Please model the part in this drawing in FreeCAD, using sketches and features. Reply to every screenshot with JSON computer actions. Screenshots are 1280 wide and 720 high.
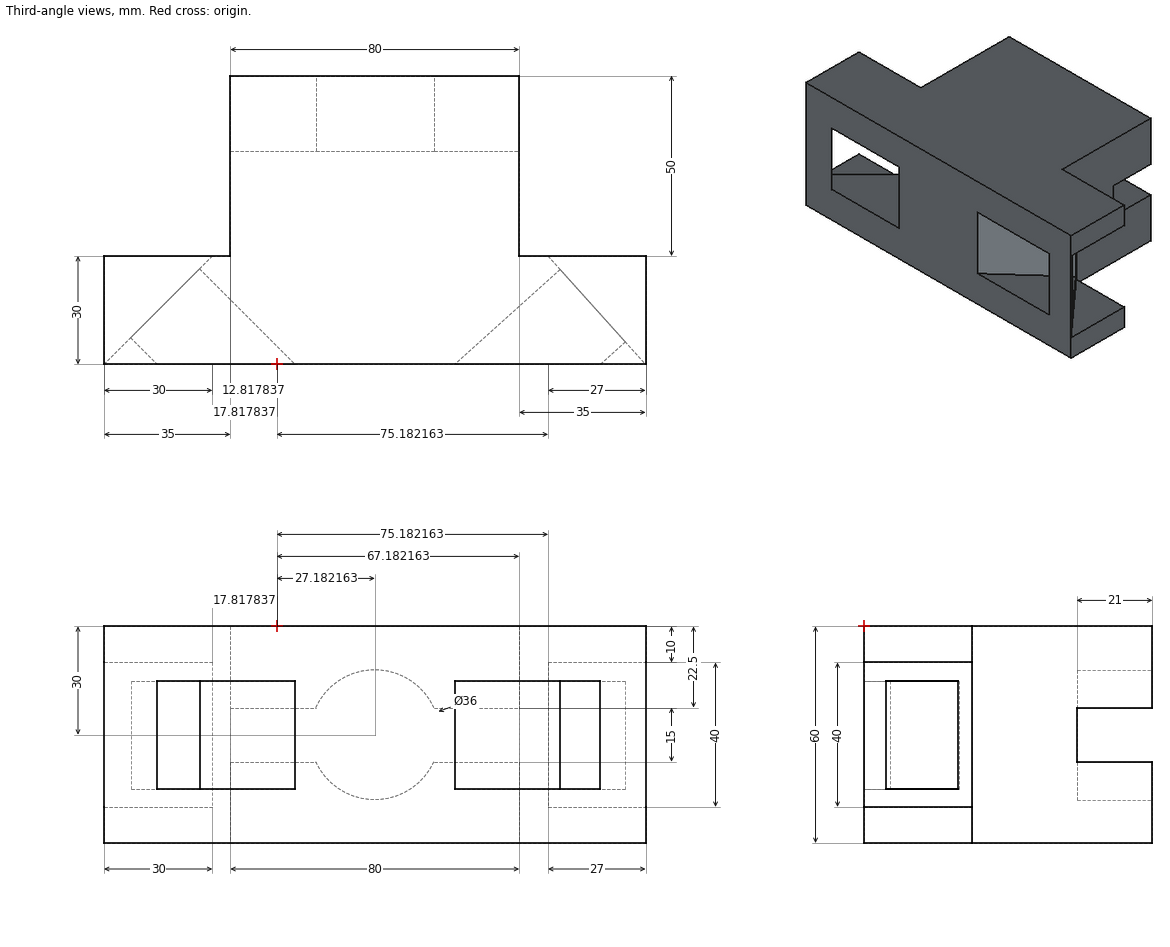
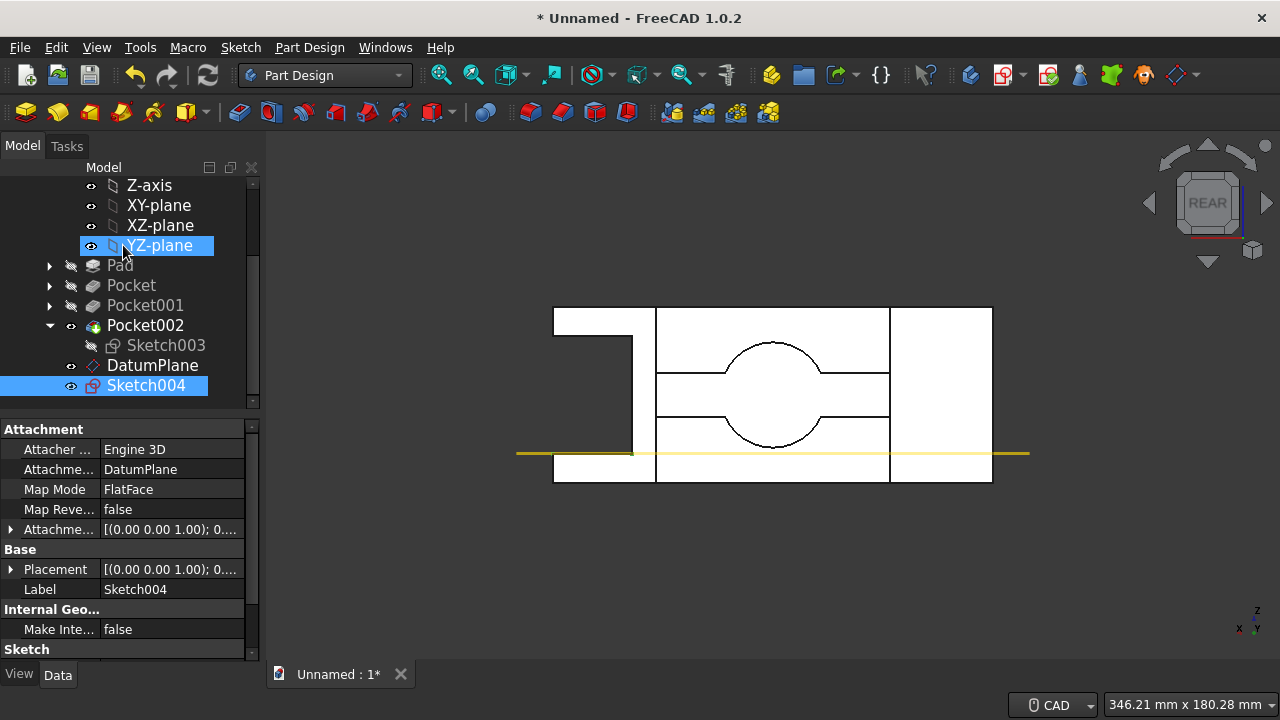
{"action": "left_click", "coordinate": [26, 112]}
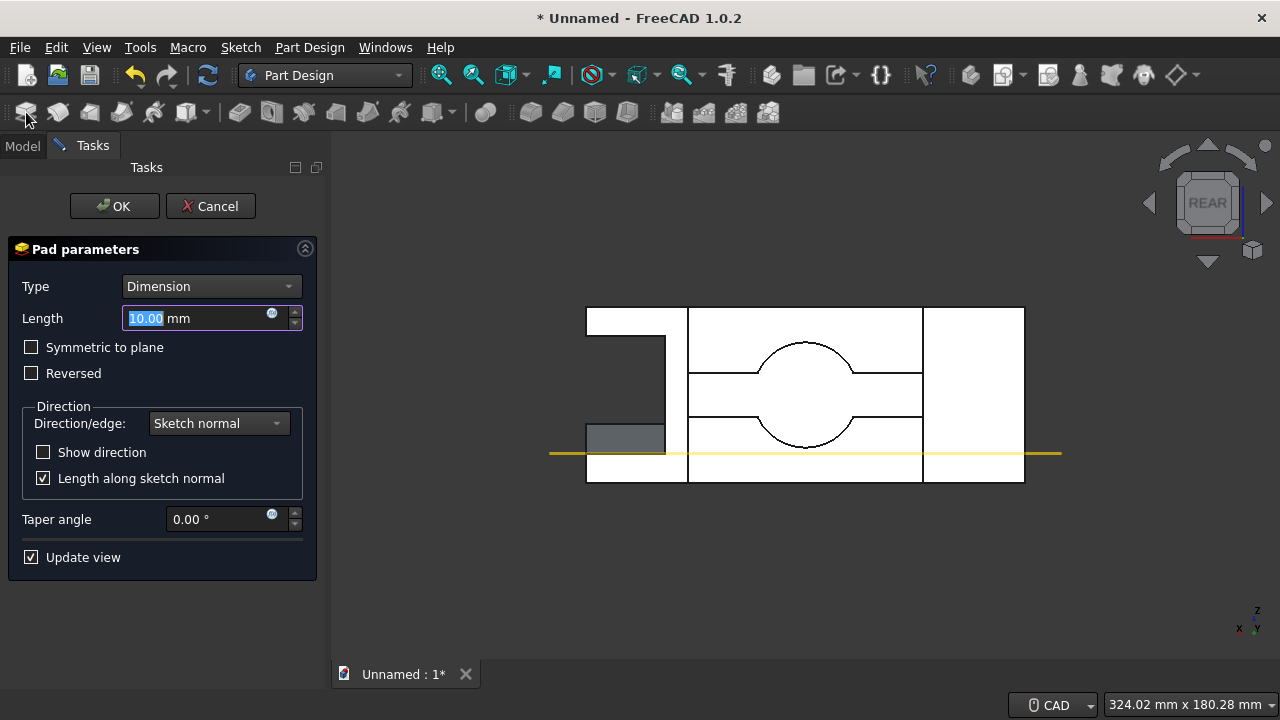
{"action": "type", "text": "40"}
{"action": "key", "text": "Tab"}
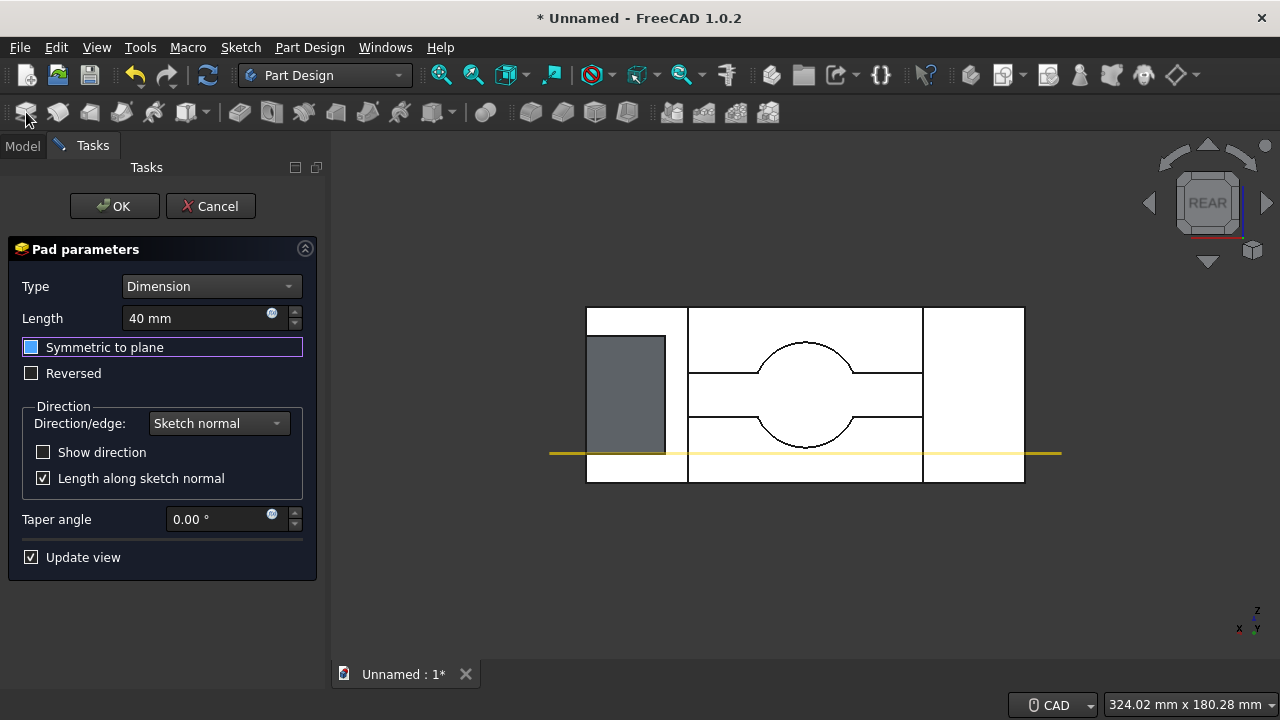
{"action": "left_click", "coordinate": [115, 206]}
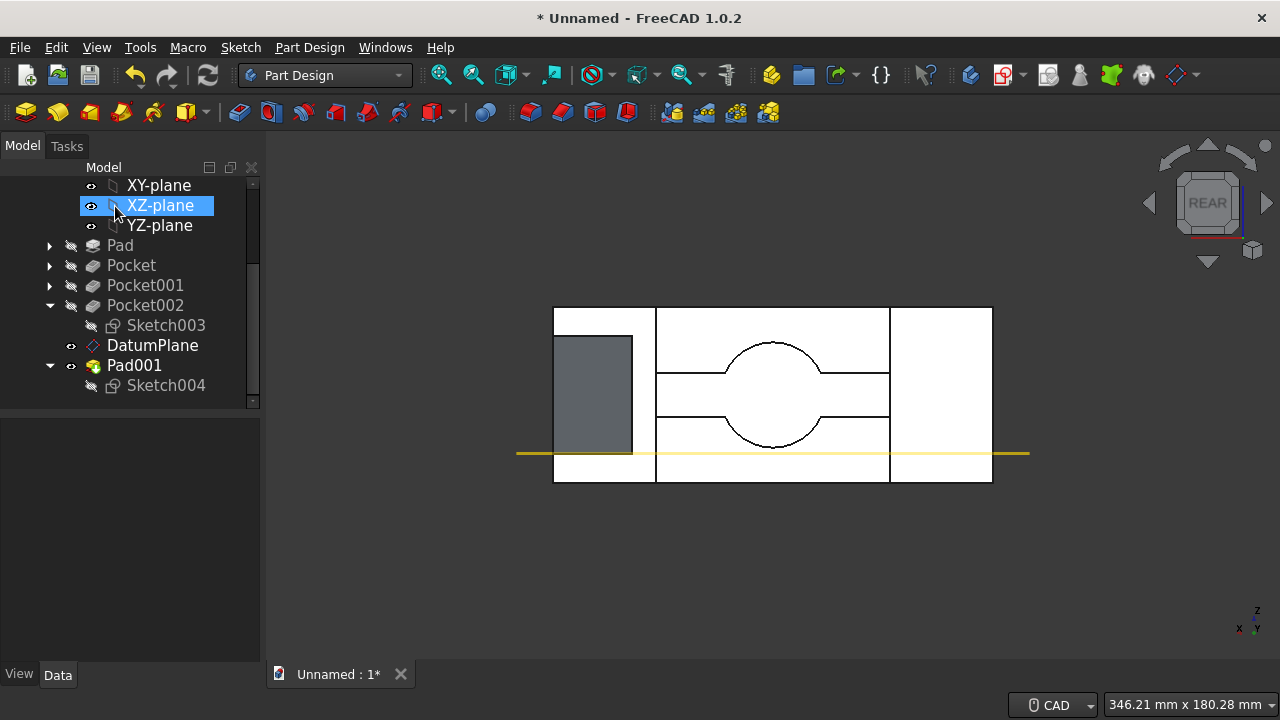
{"action": "left_click", "coordinate": [116, 346]}
{"action": "key", "text": "space"}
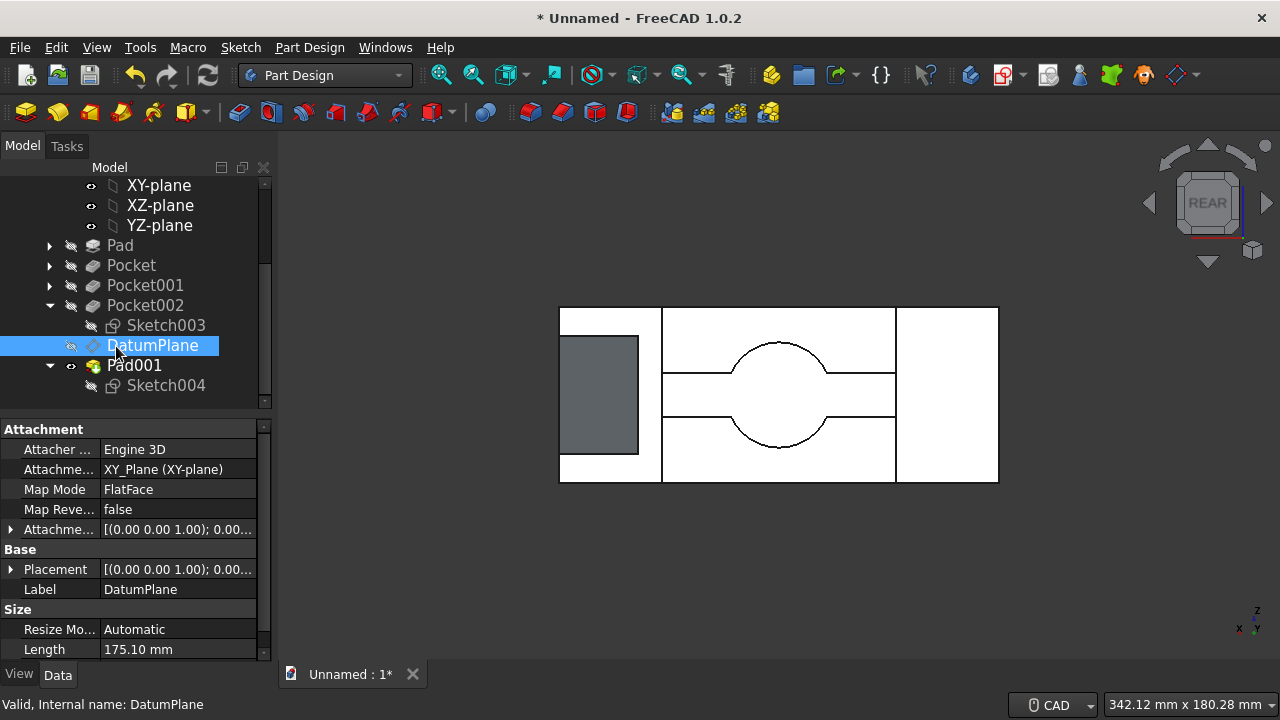
{"action": "left_click", "coordinate": [442, 76]}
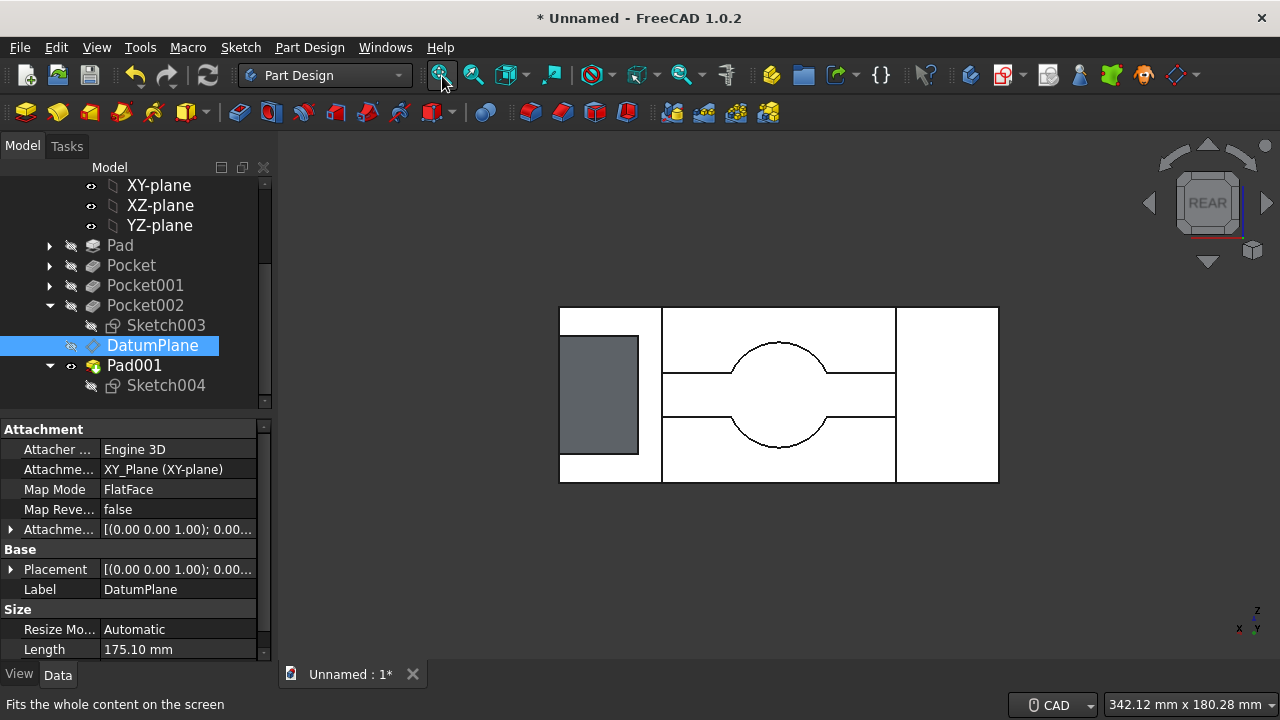
{"action": "left_click", "coordinate": [599, 394]}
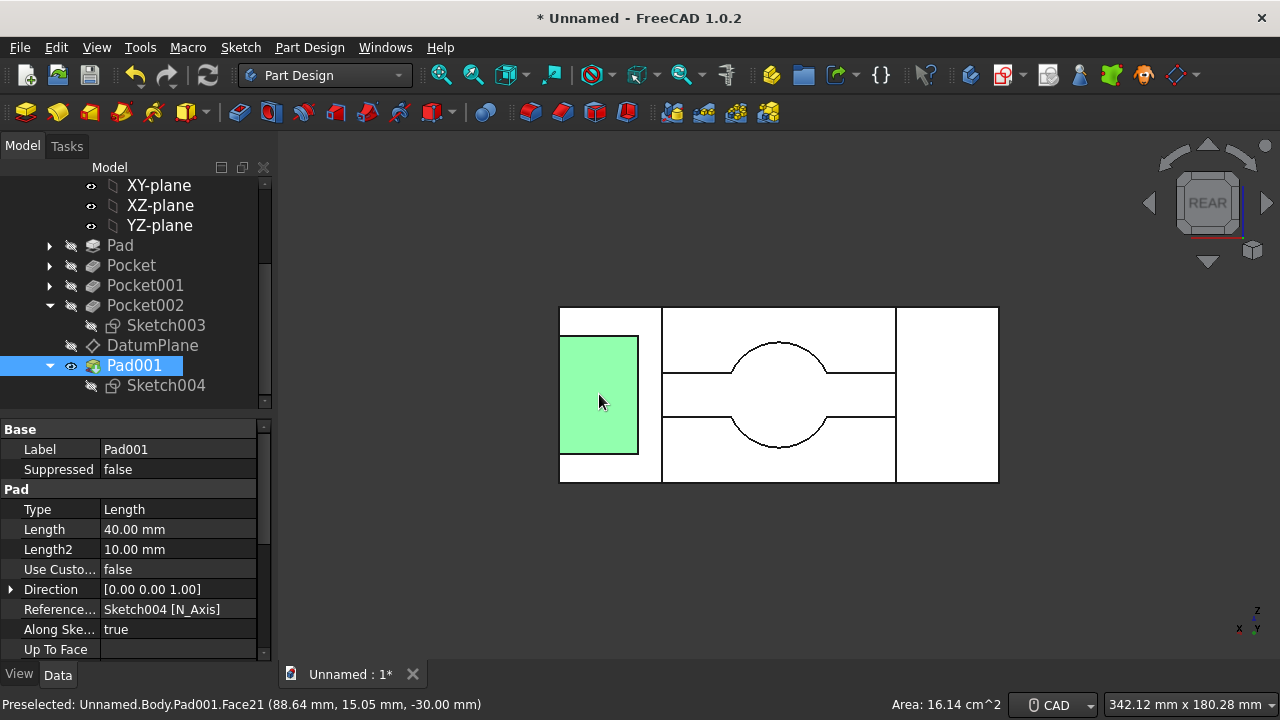
{"action": "left_click", "coordinate": [1004, 76]}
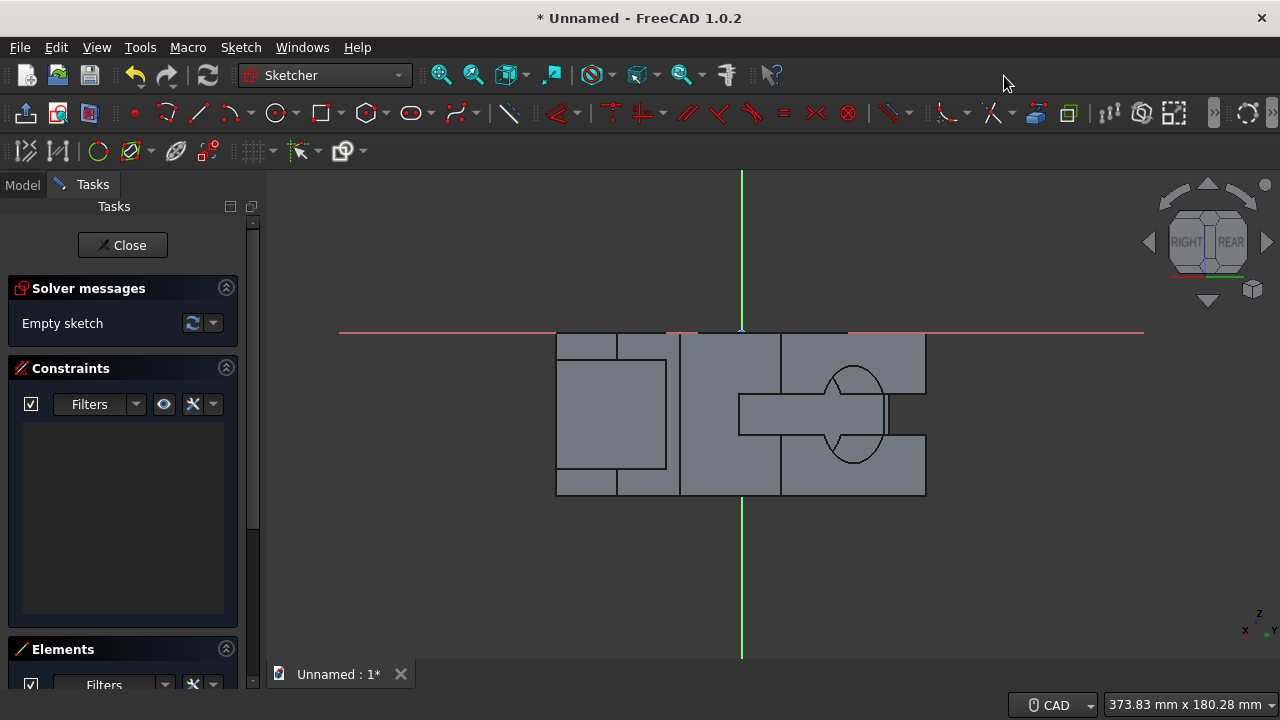
{"action": "scroll", "coordinate": [635, 382], "scroll_direction": "up", "scroll_amount": 5}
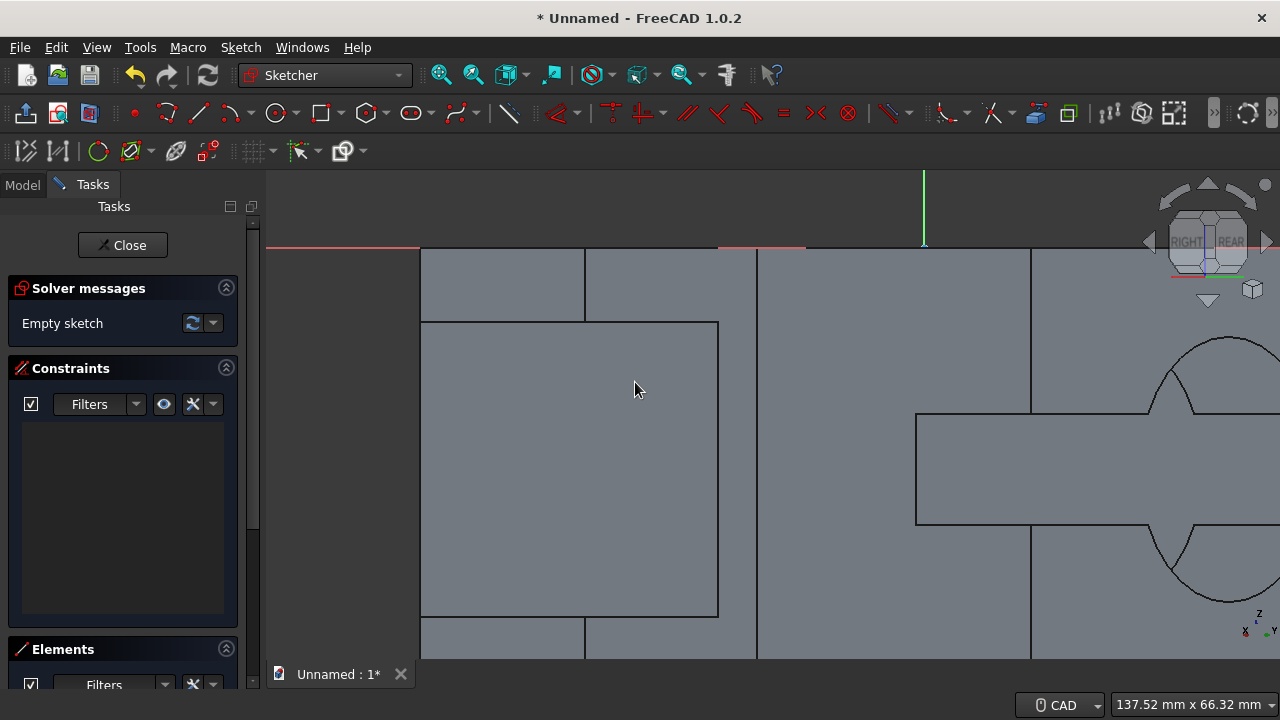
{"action": "left_click", "coordinate": [322, 114]}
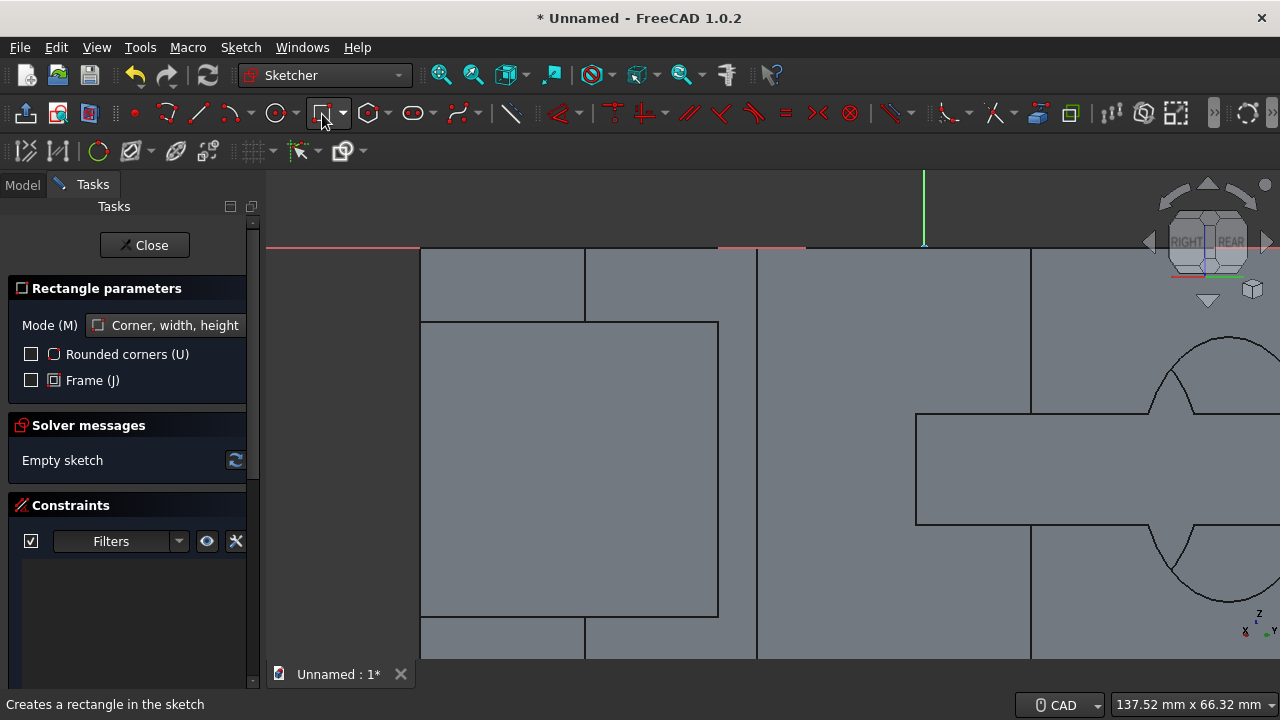
{"action": "left_click", "coordinate": [482, 359]}
{"action": "left_click", "coordinate": [681, 580]}
{"action": "key", "text": "Escape"}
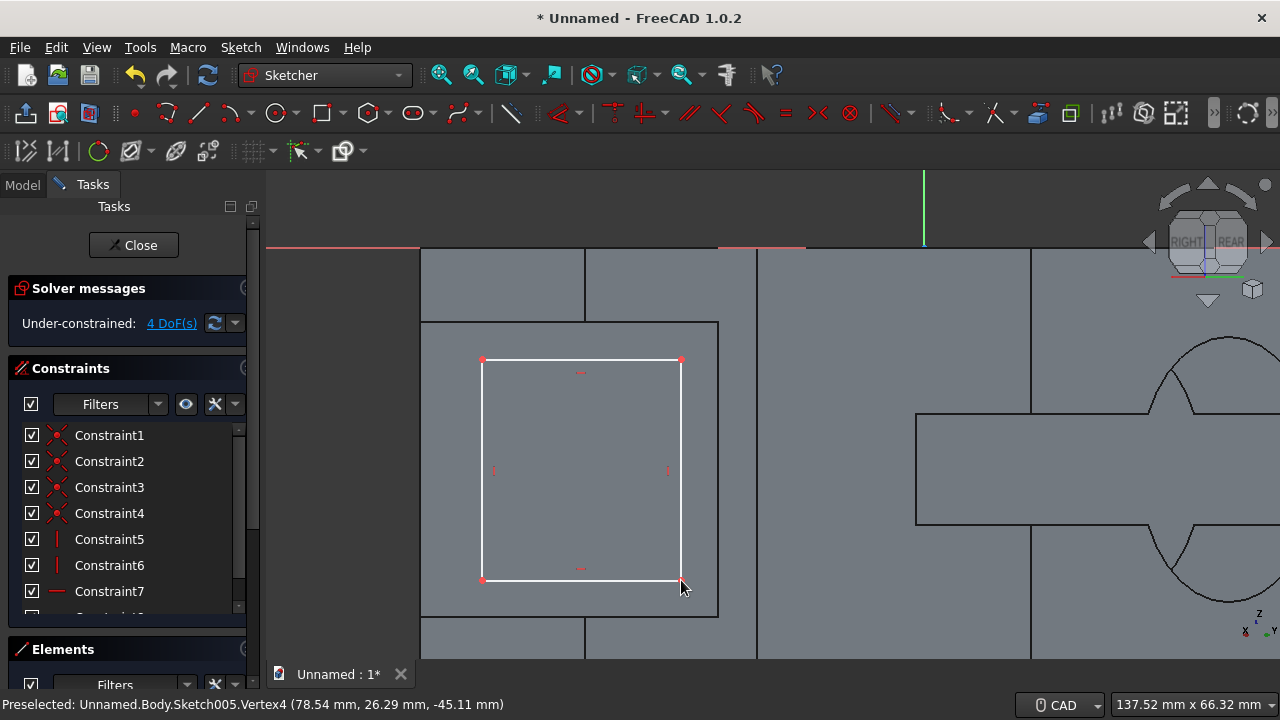
{"action": "left_click", "coordinate": [558, 114]}